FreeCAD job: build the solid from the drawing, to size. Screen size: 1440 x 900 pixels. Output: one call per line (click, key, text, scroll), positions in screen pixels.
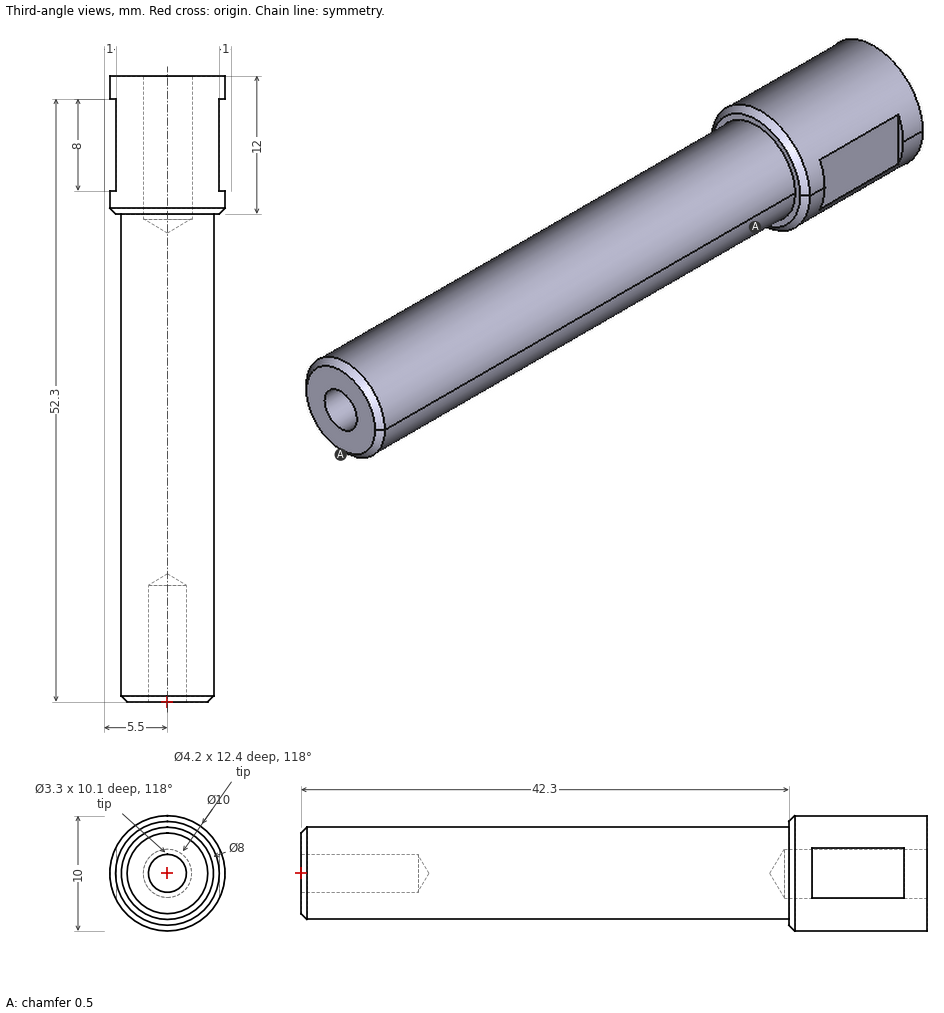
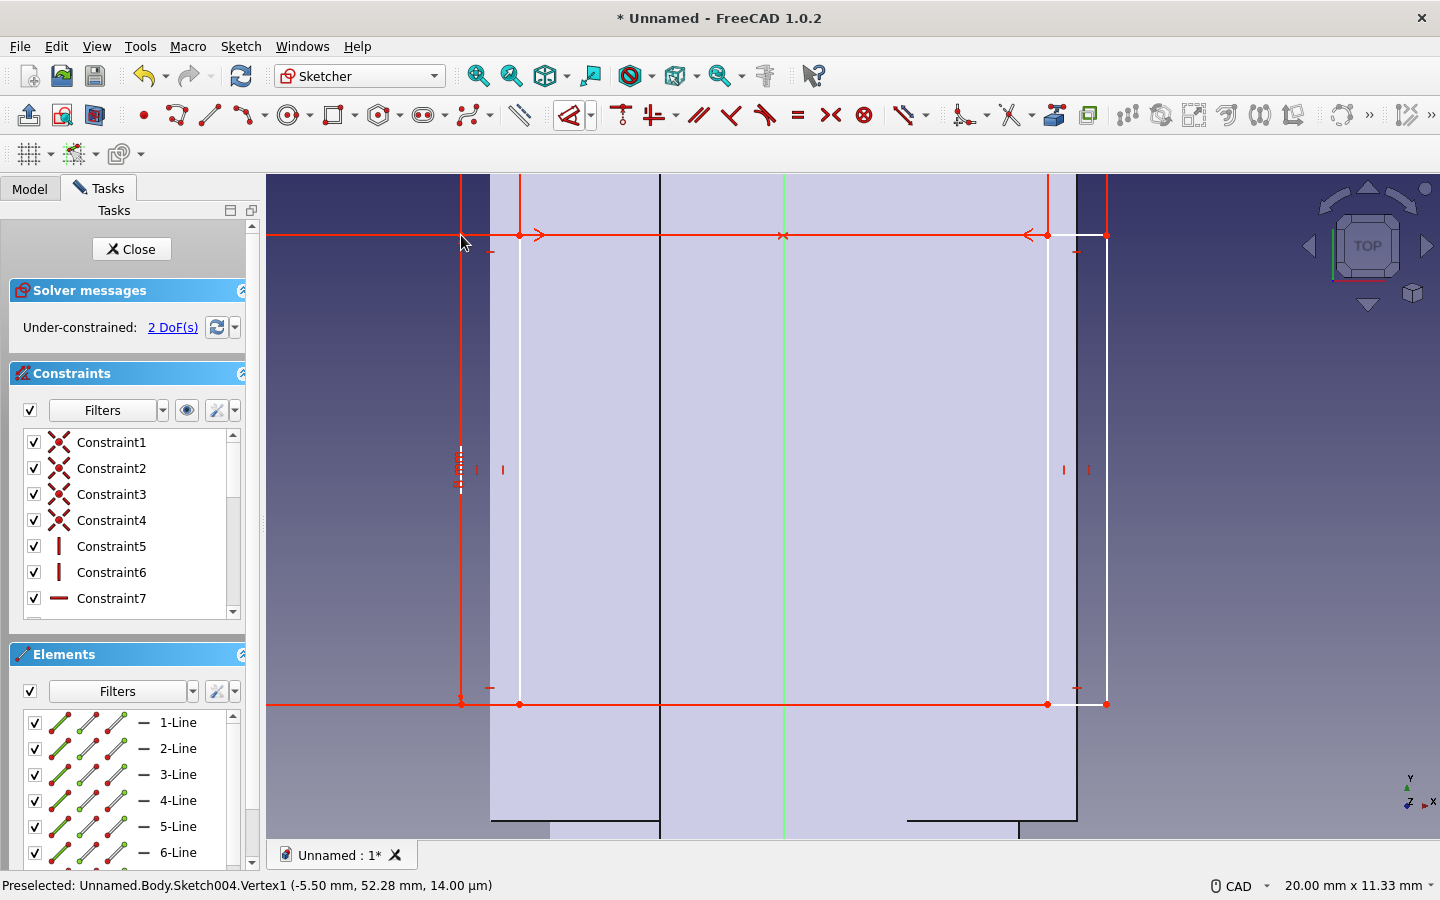
click(461, 235)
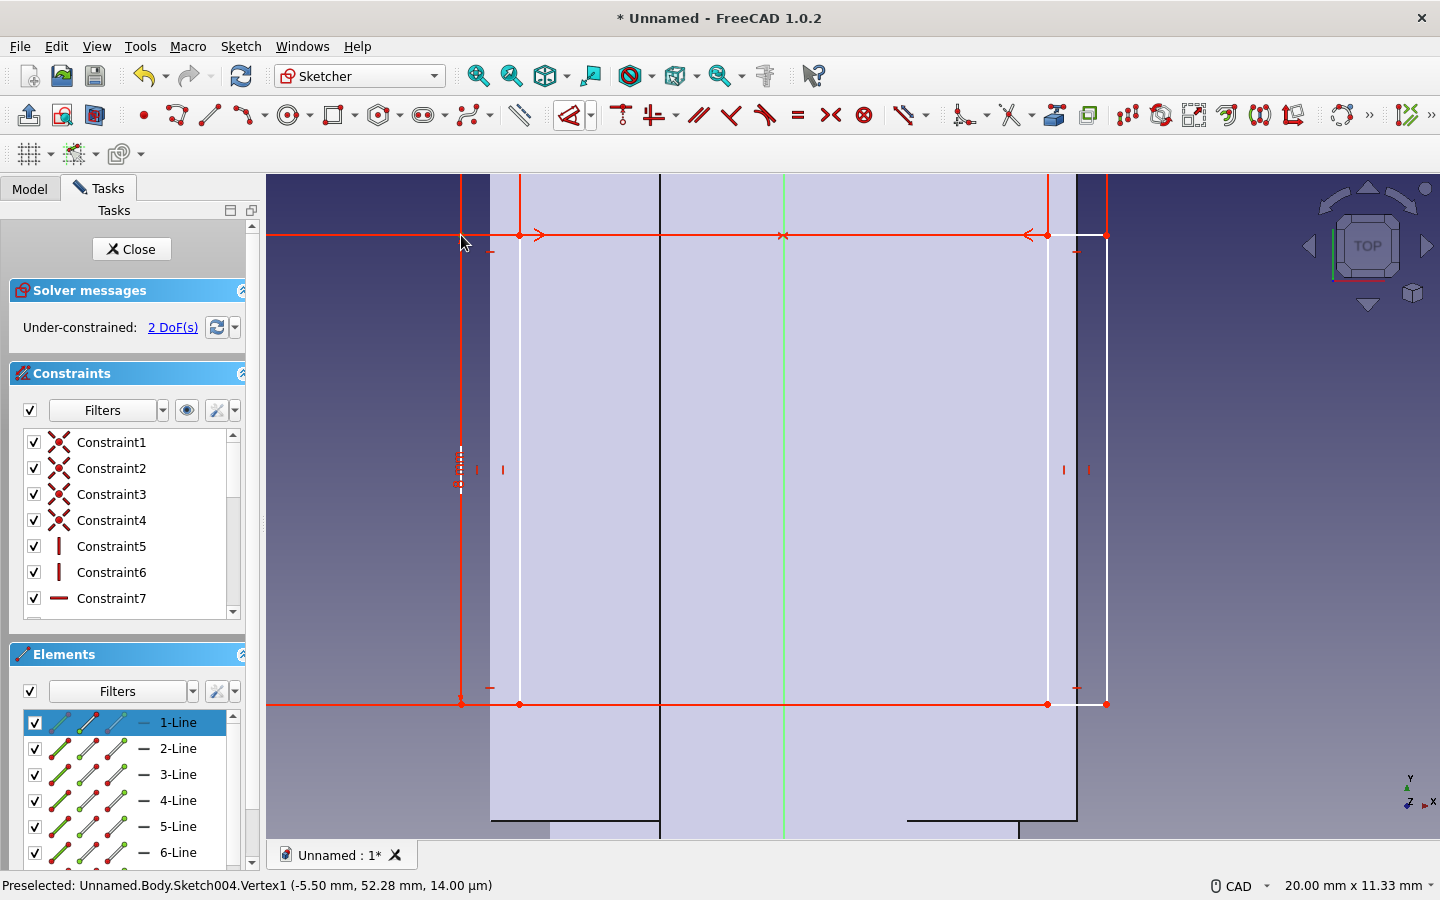
click(590, 116)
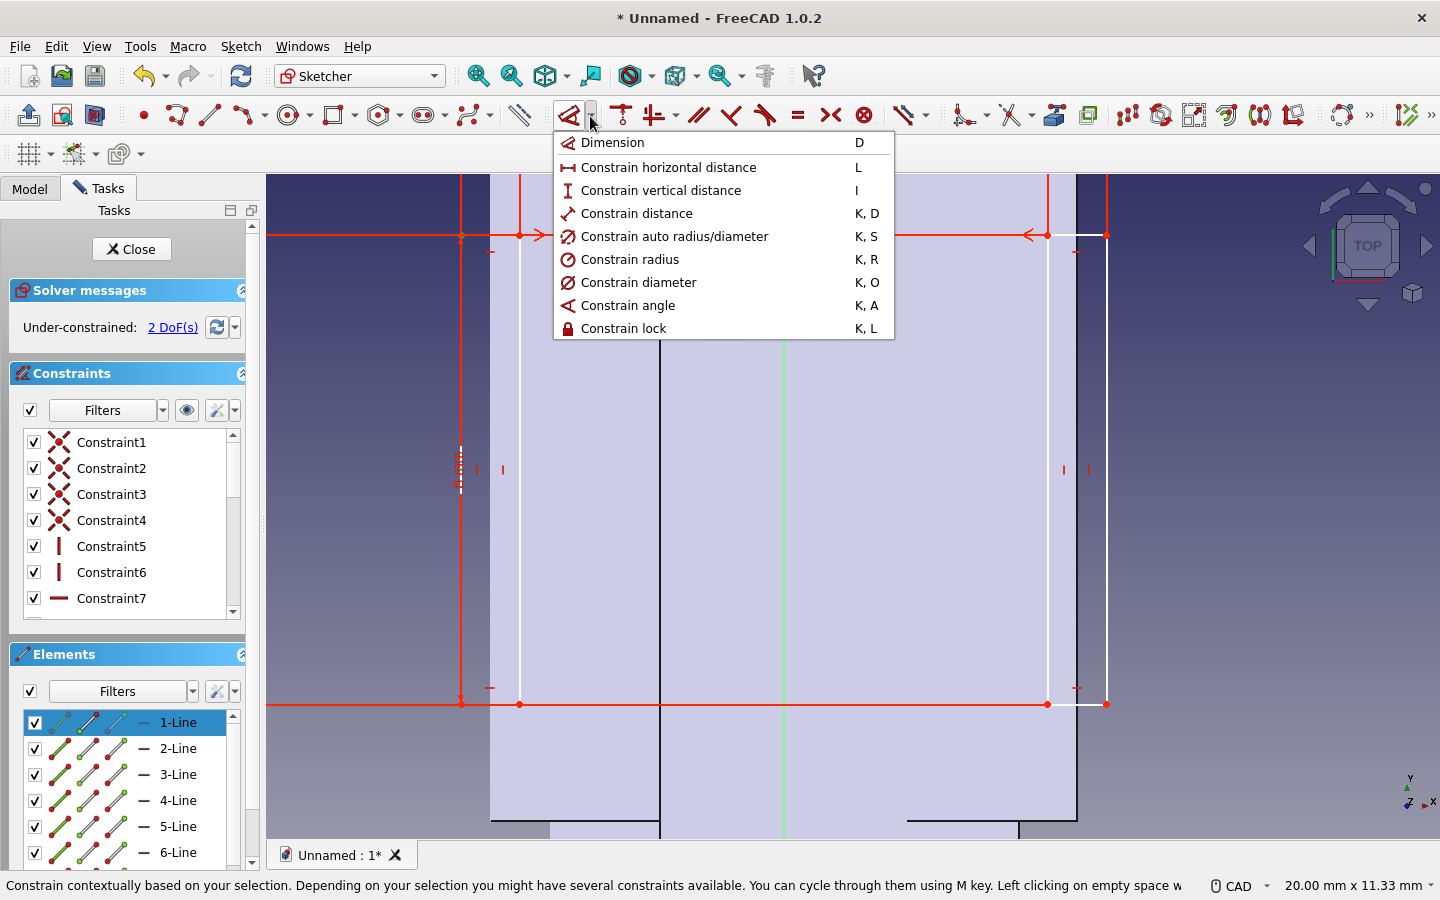
click(724, 168)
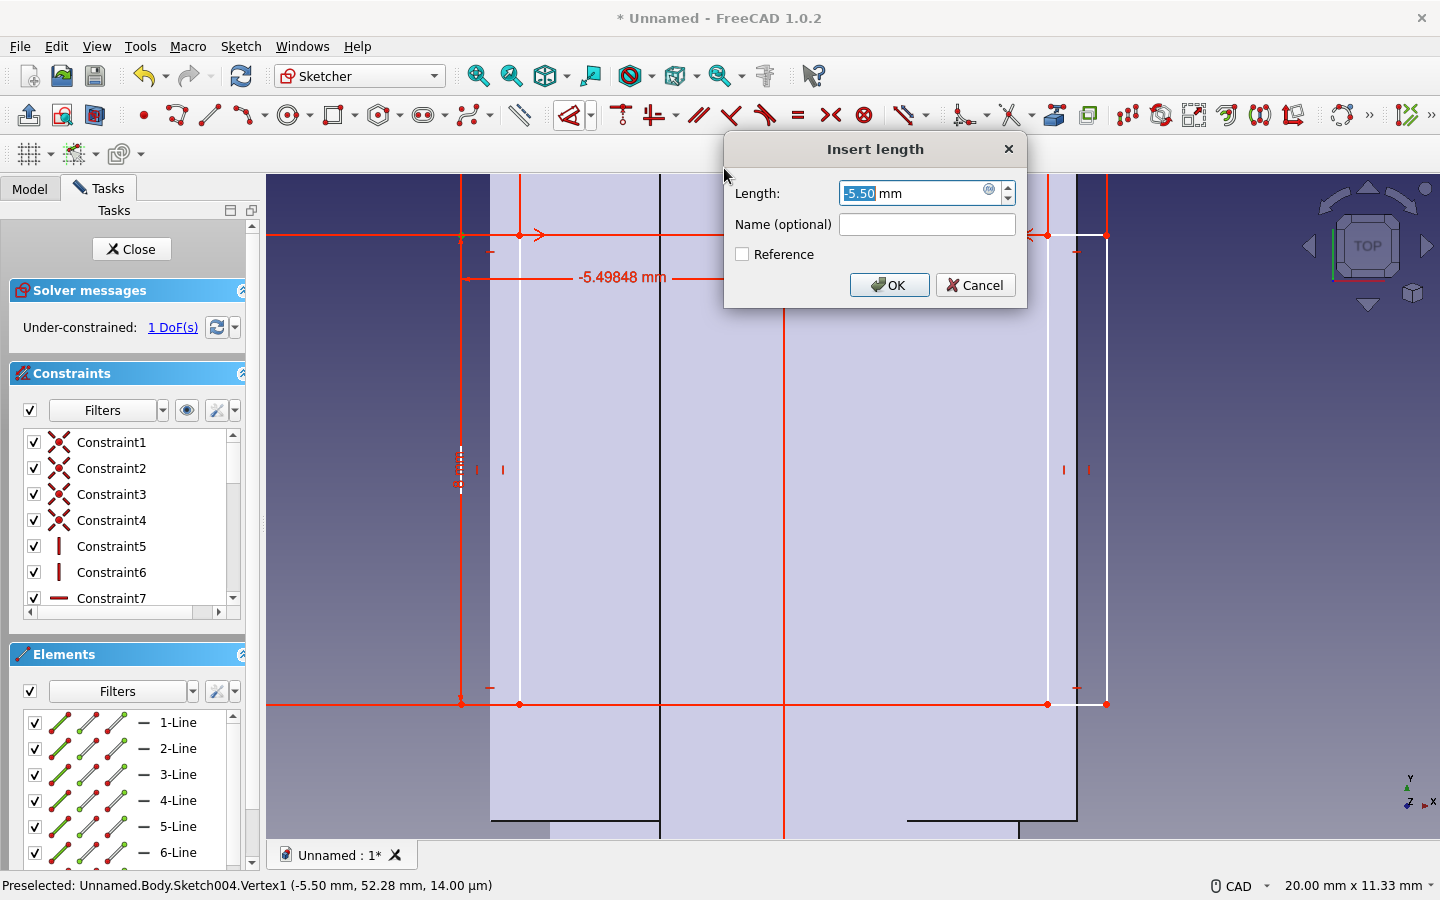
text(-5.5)
key(Return)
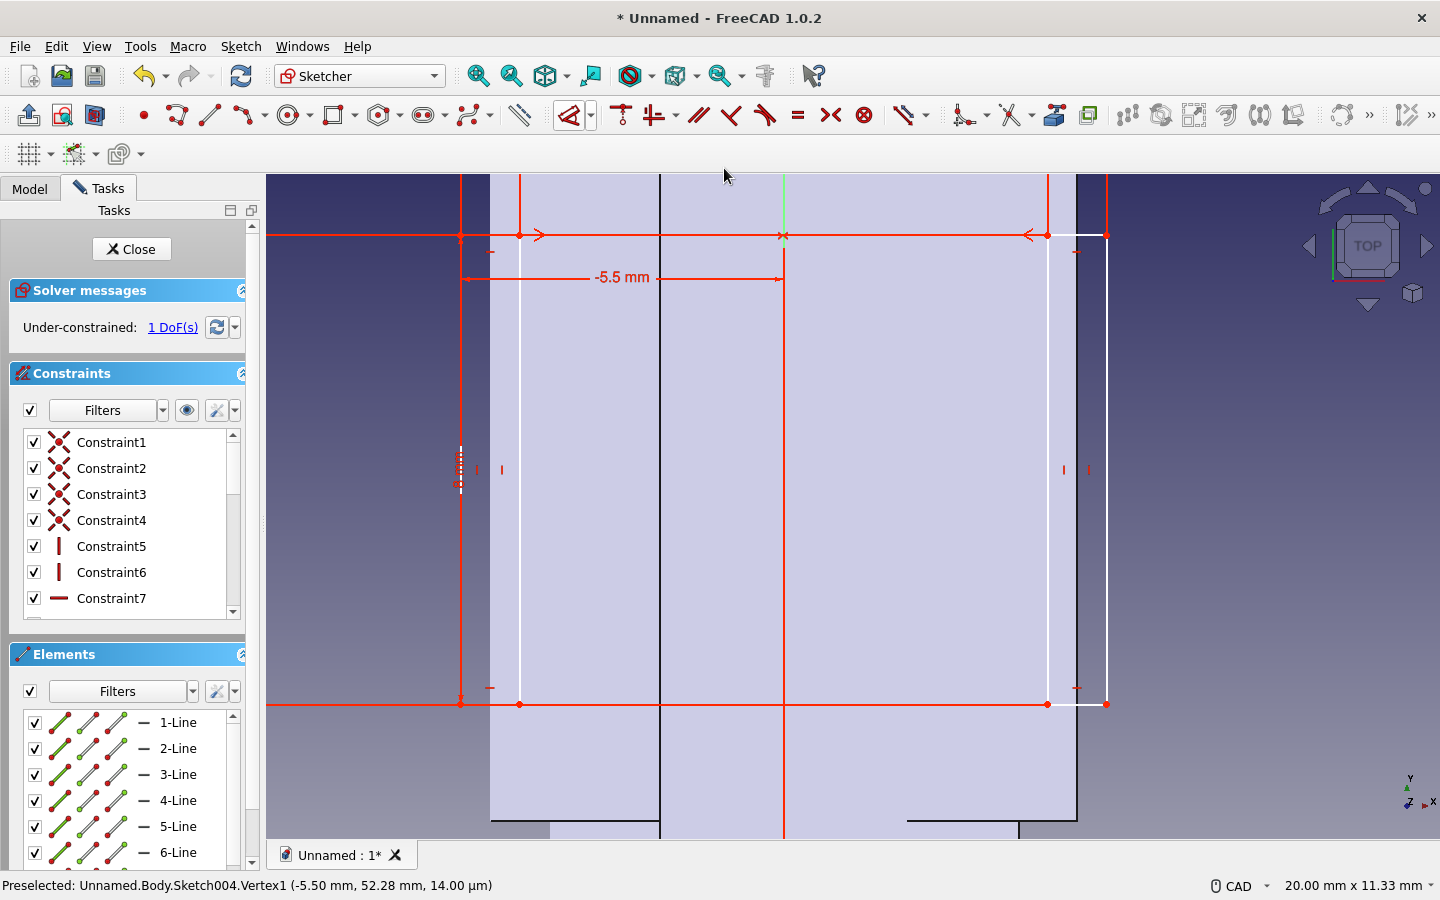
click(461, 235)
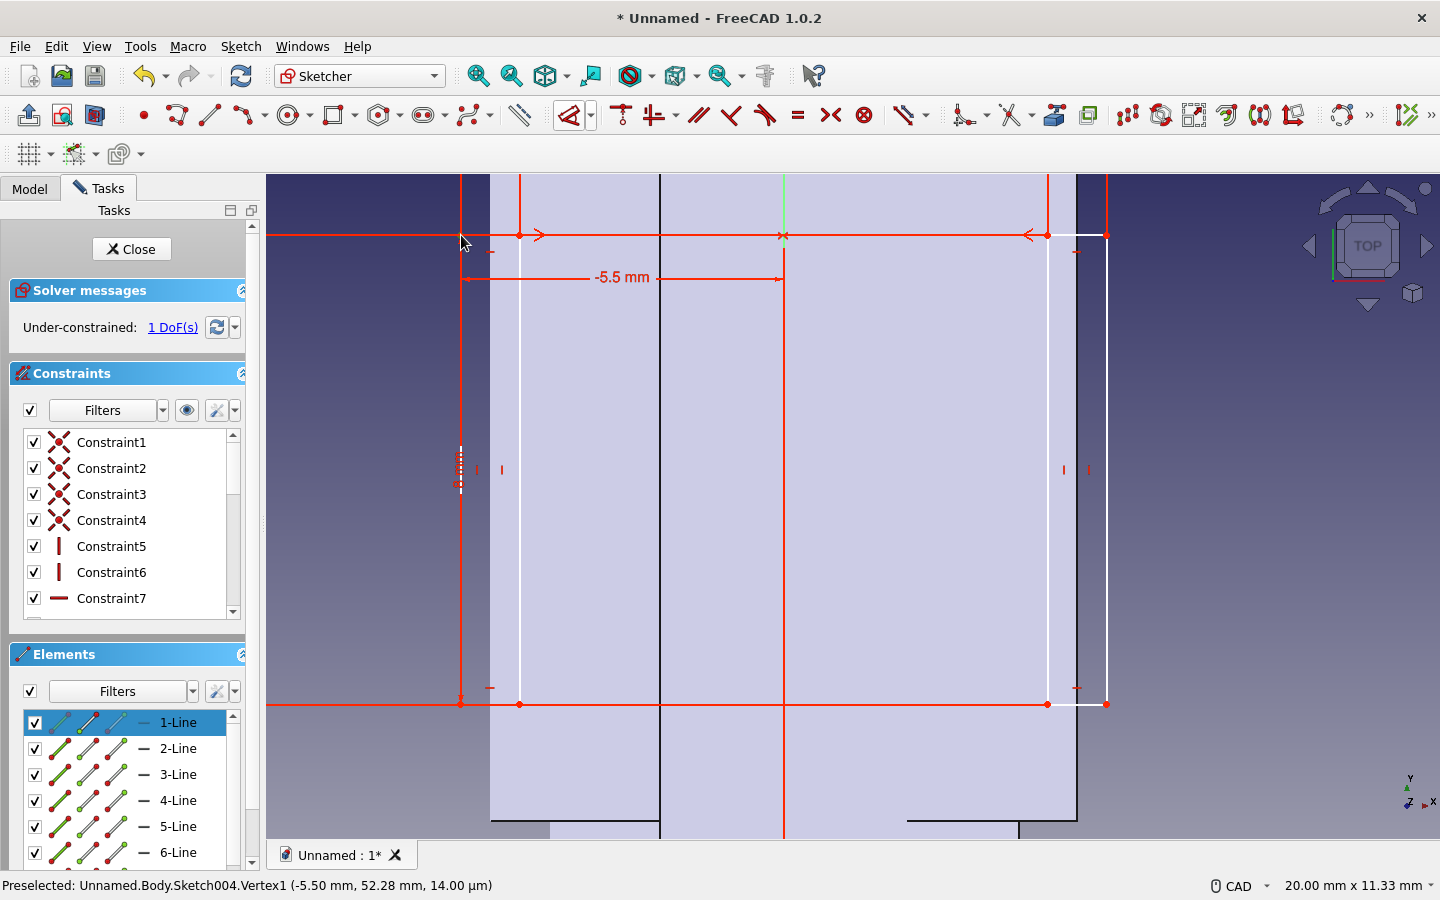
key(i)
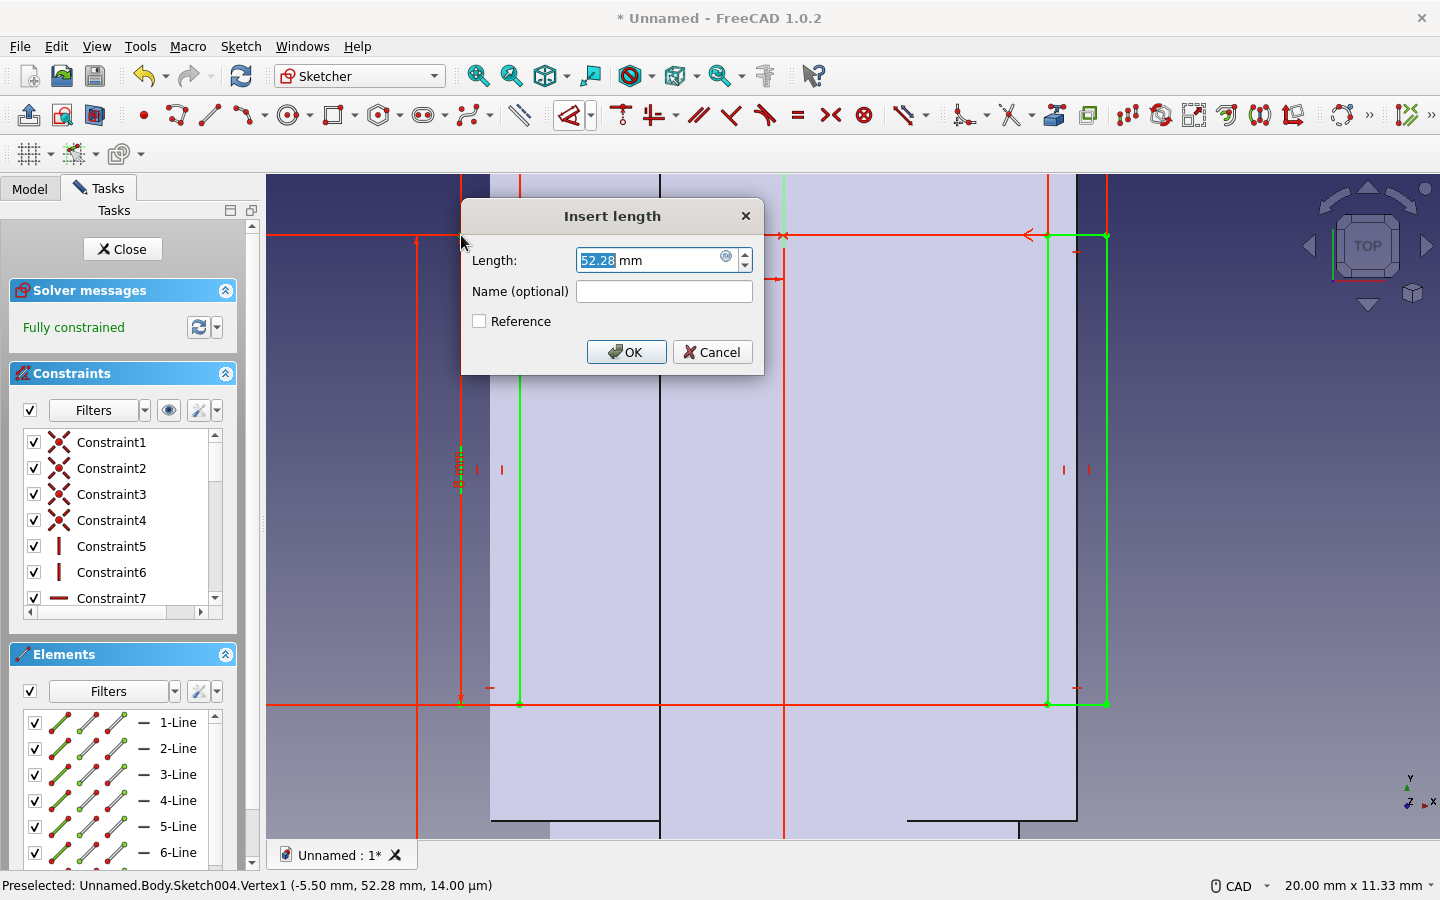
text(52.3)
key(Return)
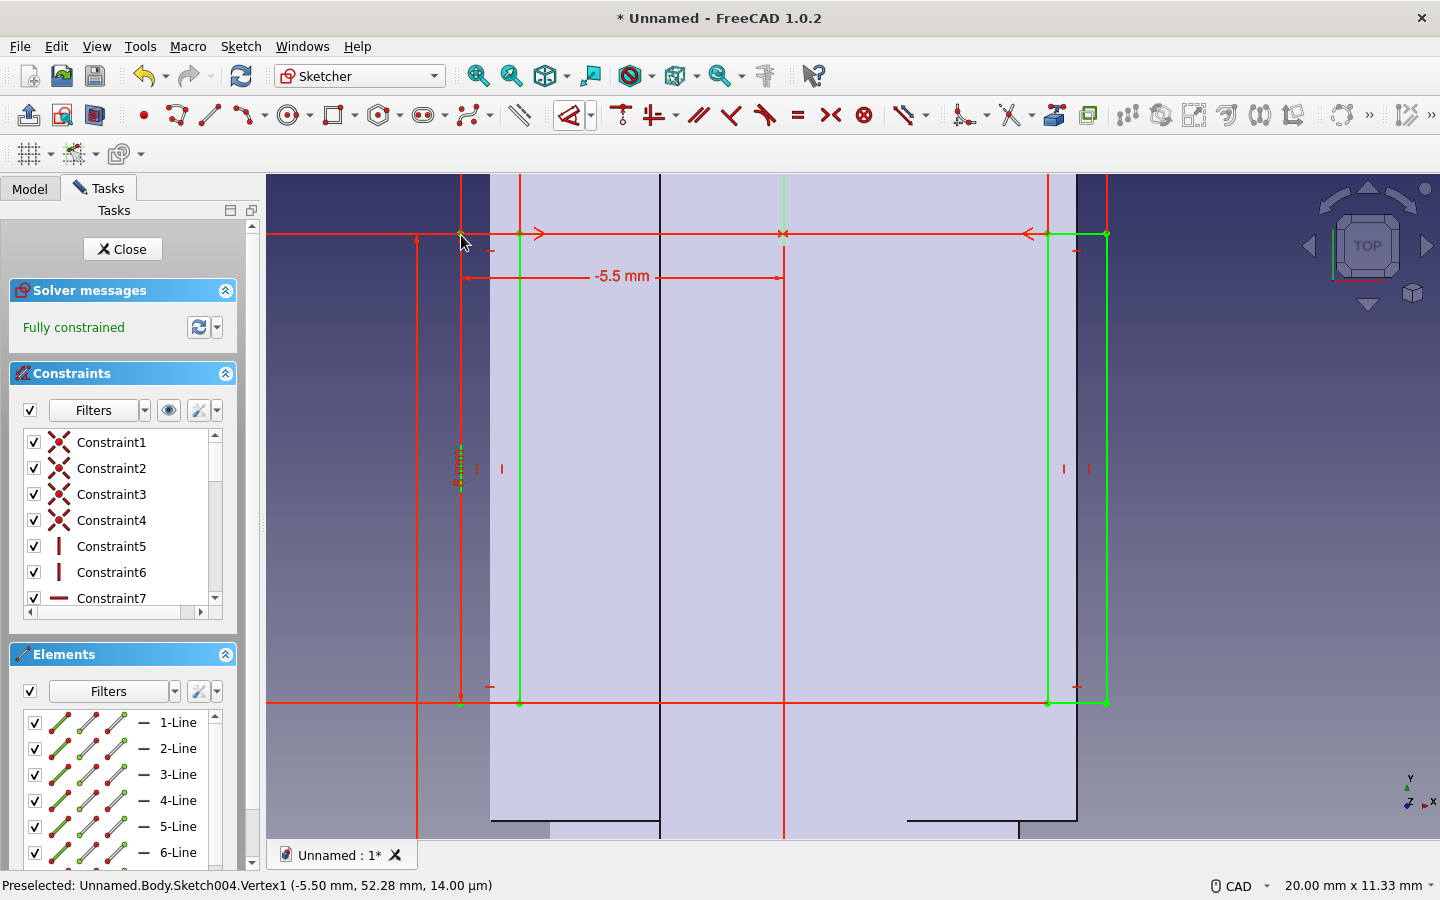
click(123, 249)